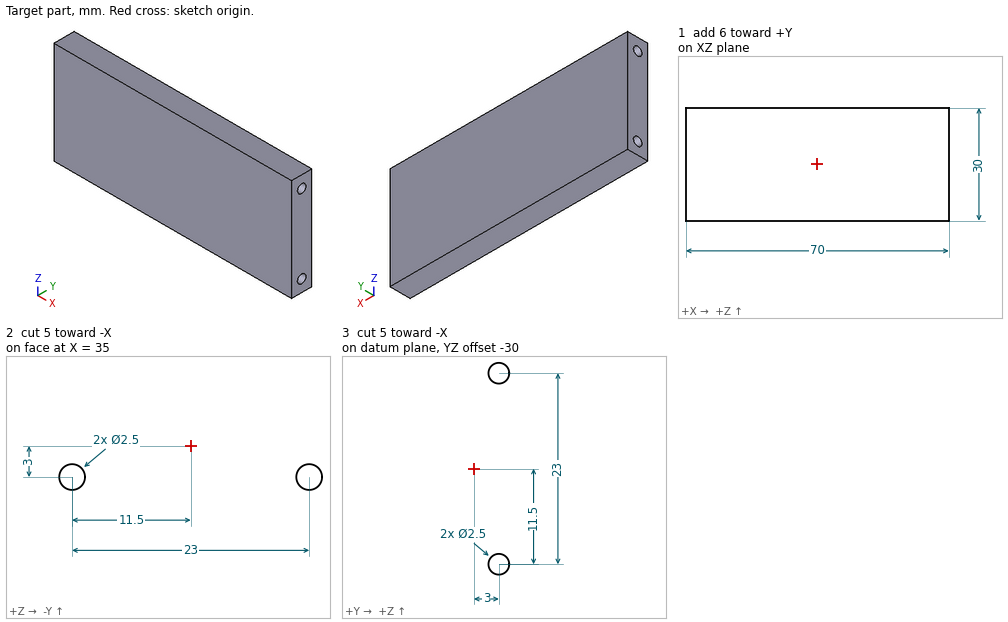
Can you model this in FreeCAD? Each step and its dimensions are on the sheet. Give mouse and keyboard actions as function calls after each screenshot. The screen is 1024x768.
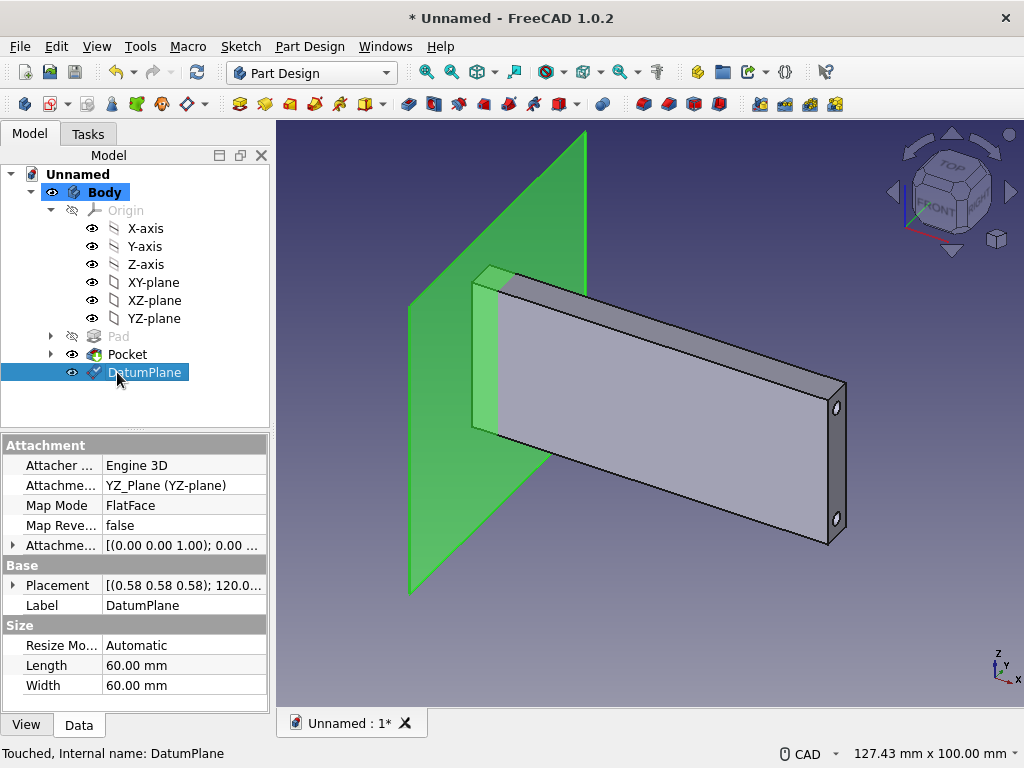
click(50, 104)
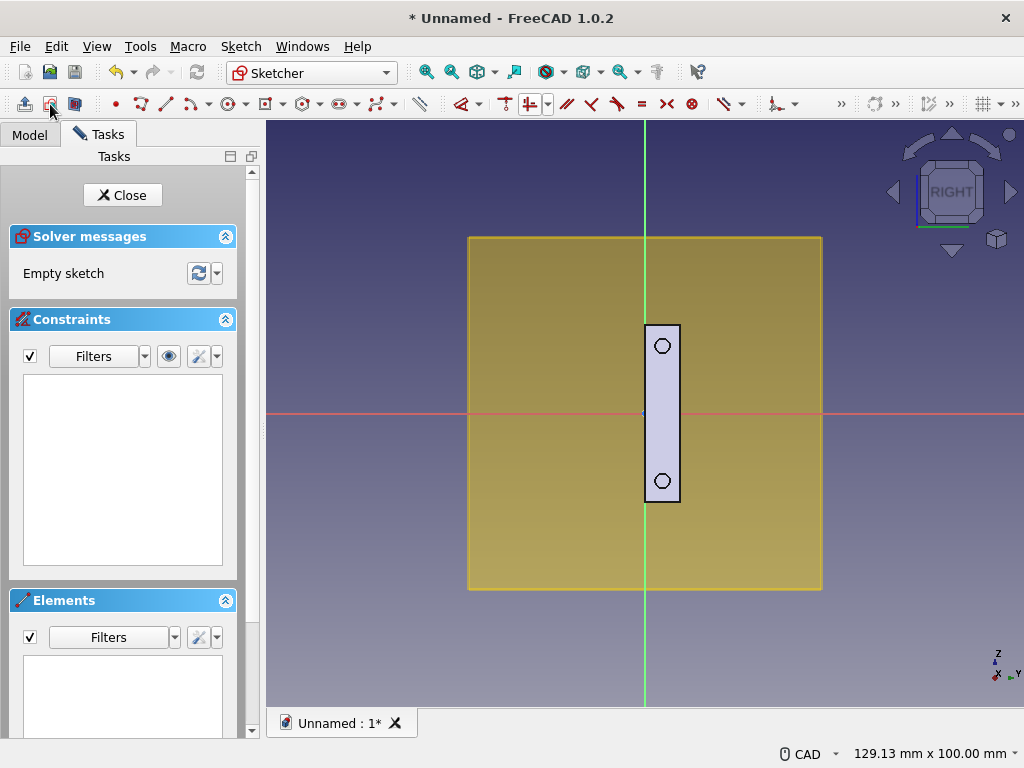
key(q)
key(s)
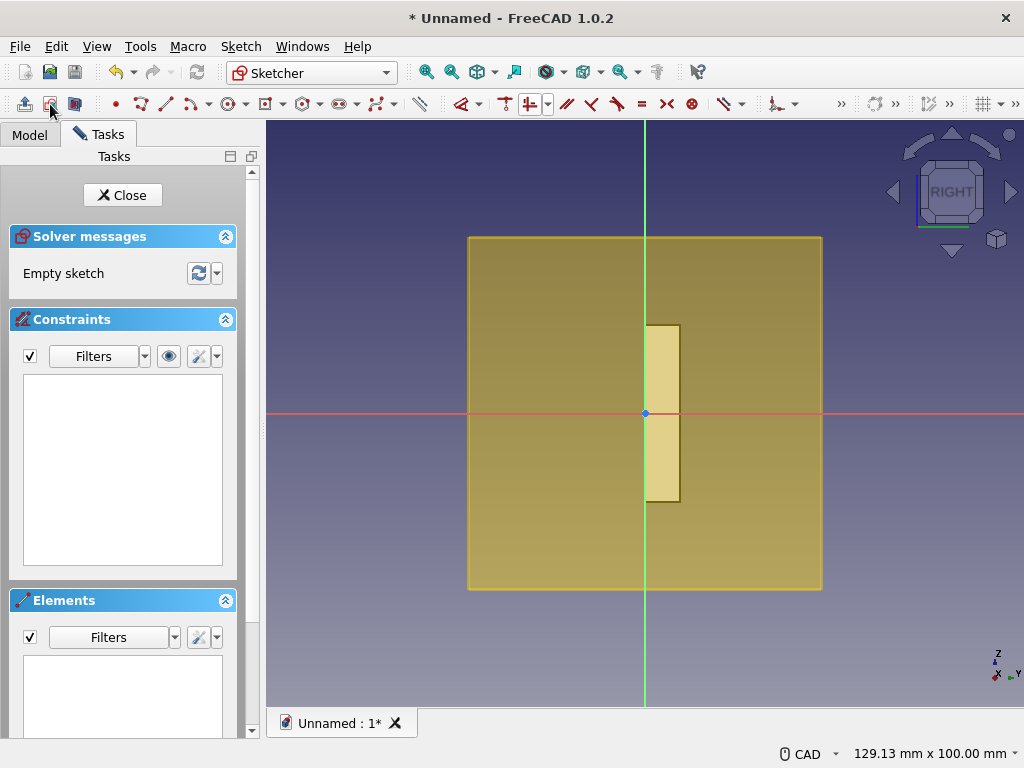
scroll(705, 414, up, 5)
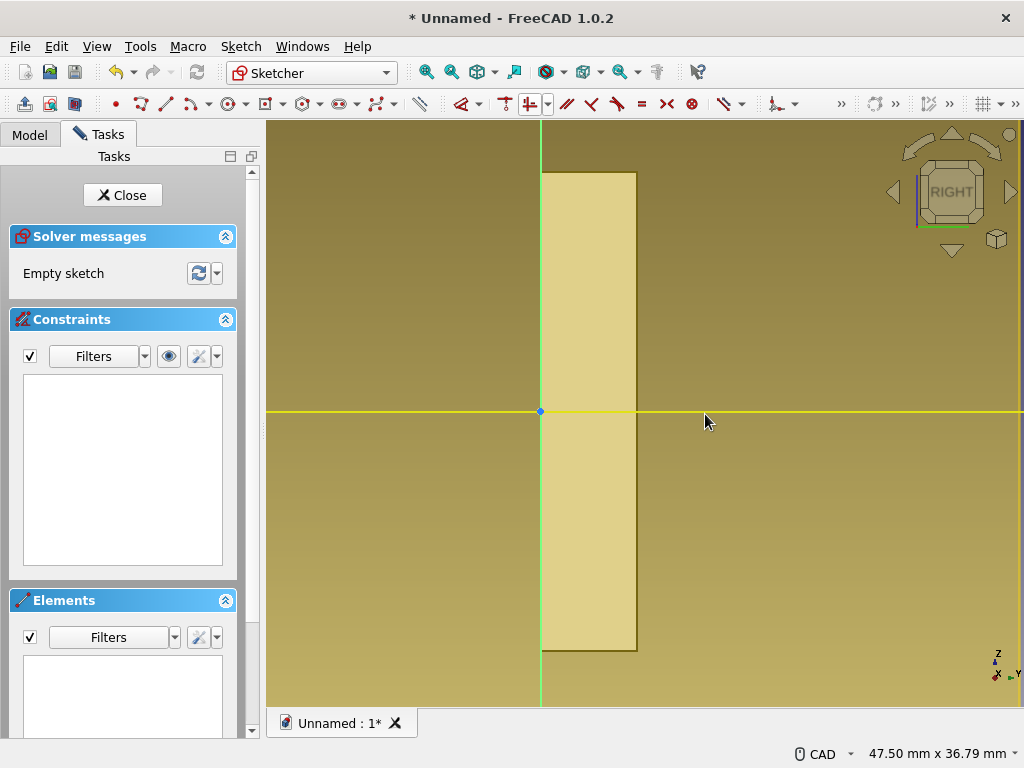
click(228, 104)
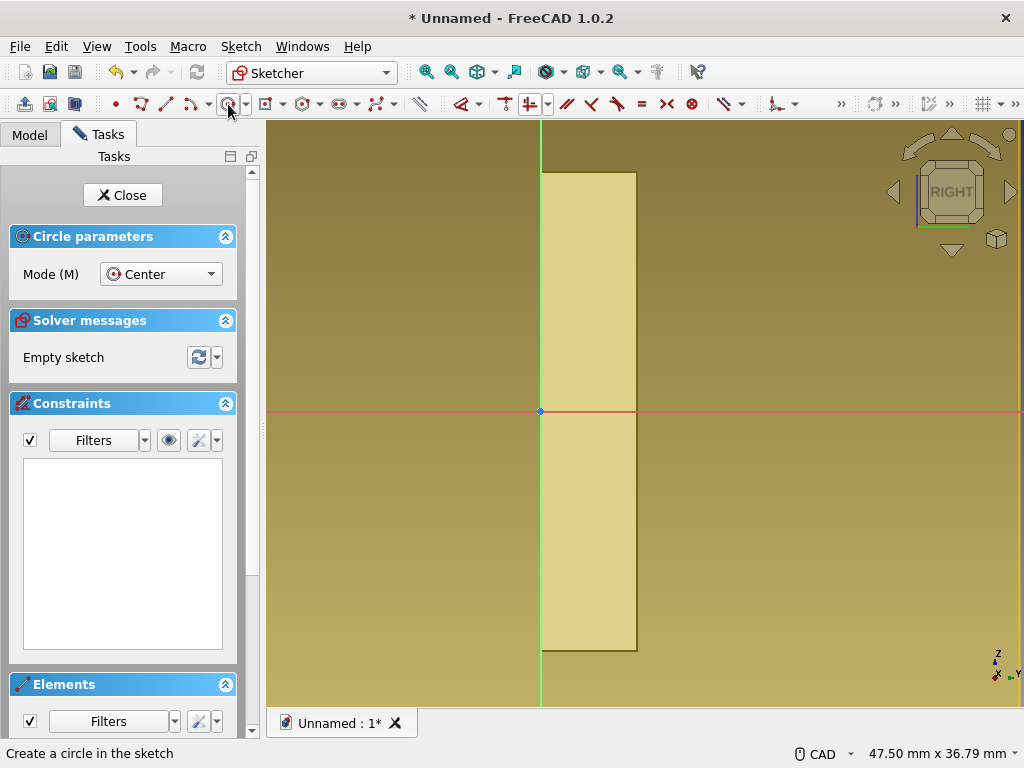
click(589, 595)
click(603, 581)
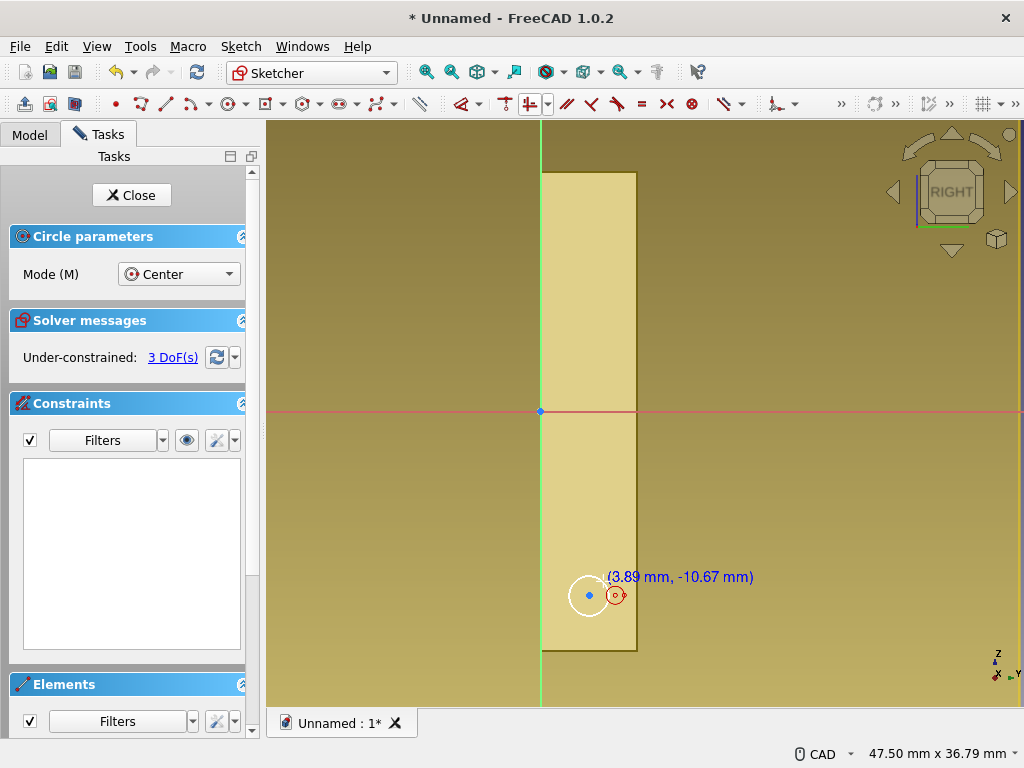
click(589, 228)
click(603, 214)
key(Escape)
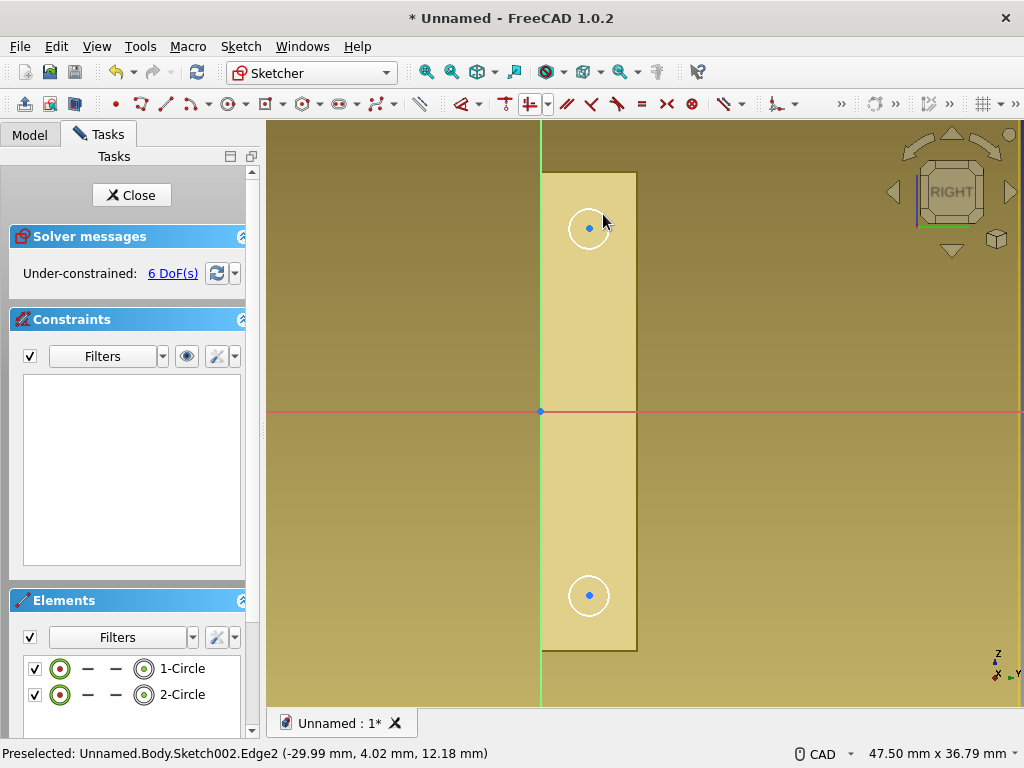
click(603, 582)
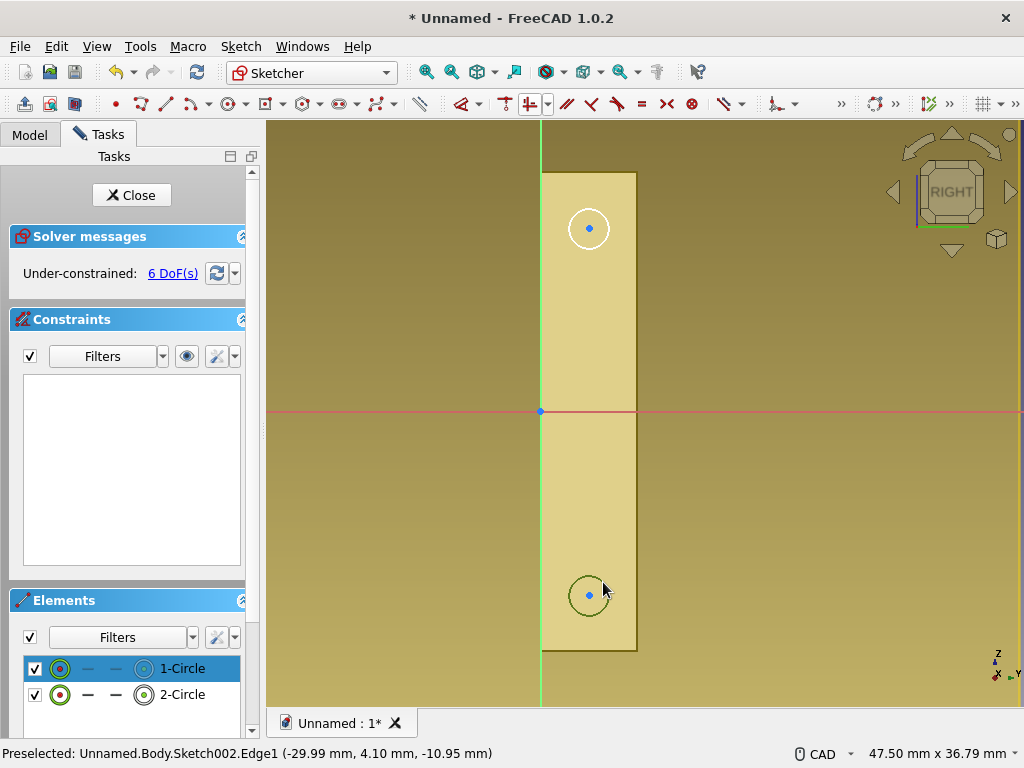
click(603, 215)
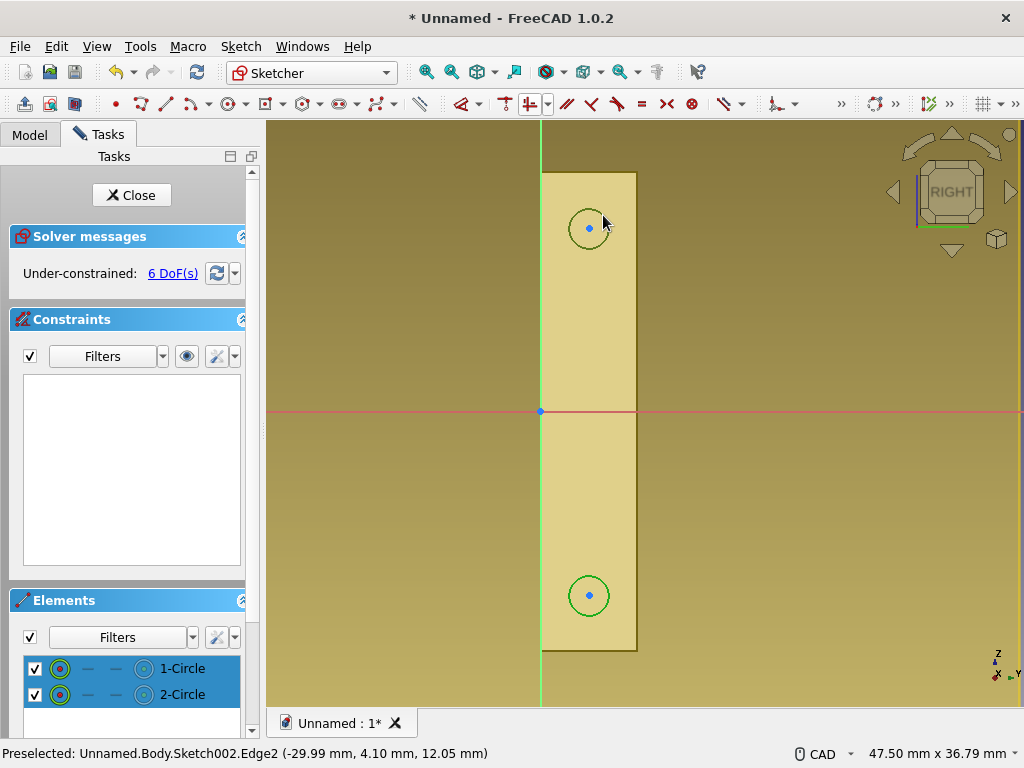
click(642, 104)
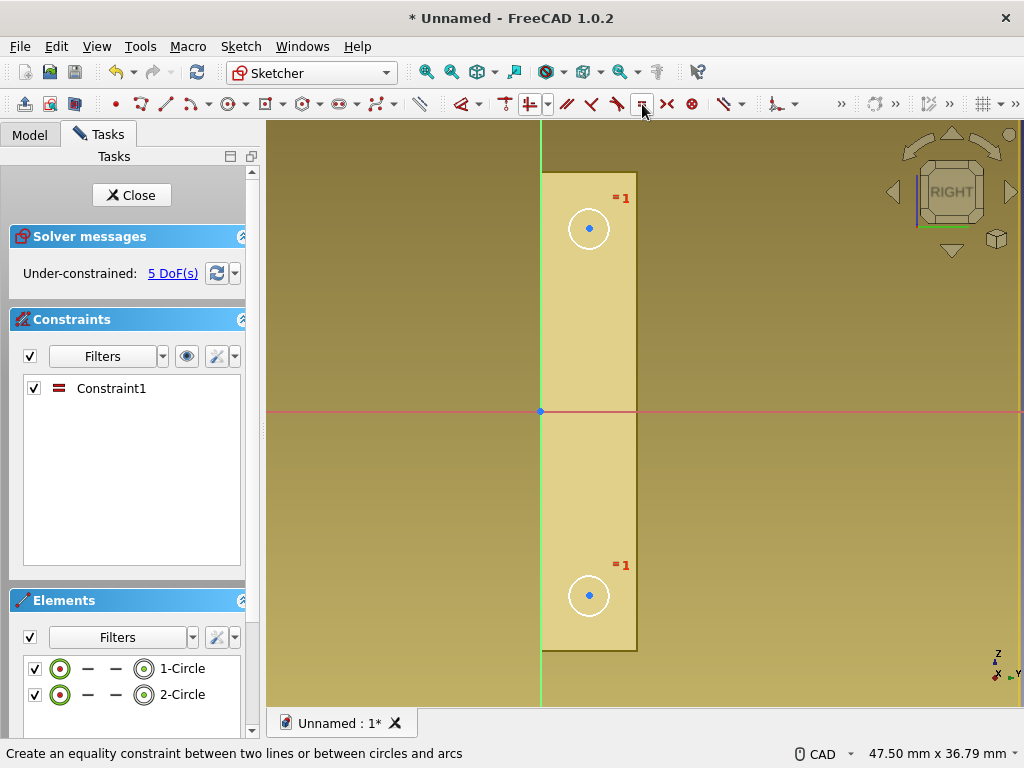
click(589, 596)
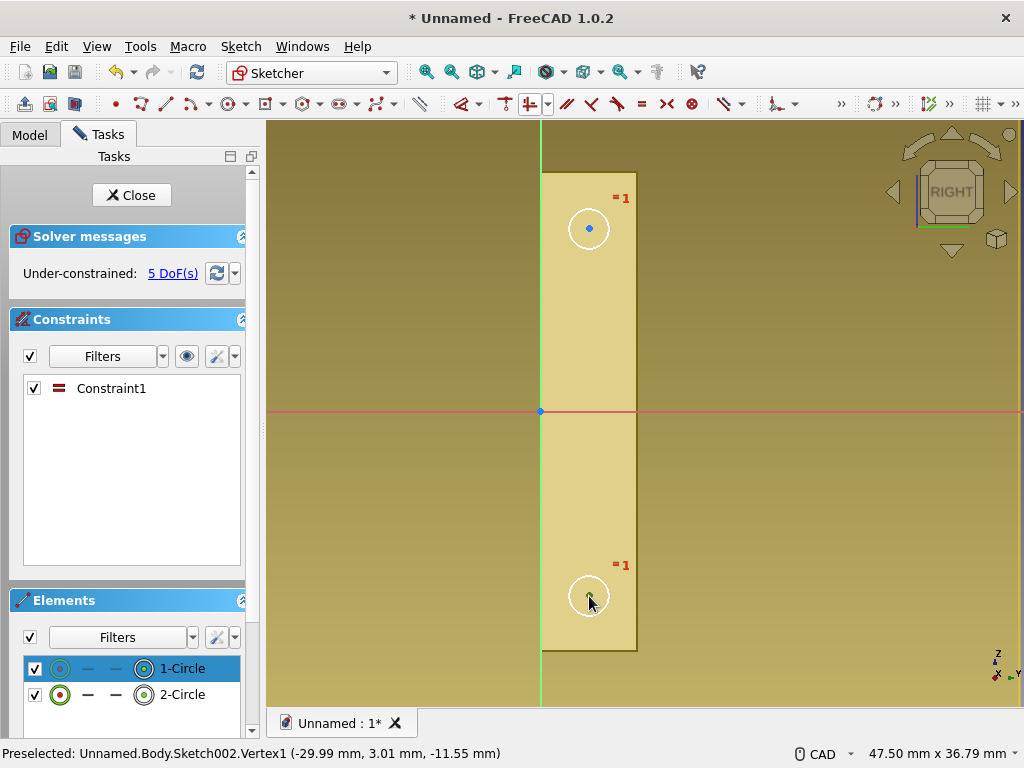
click(589, 229)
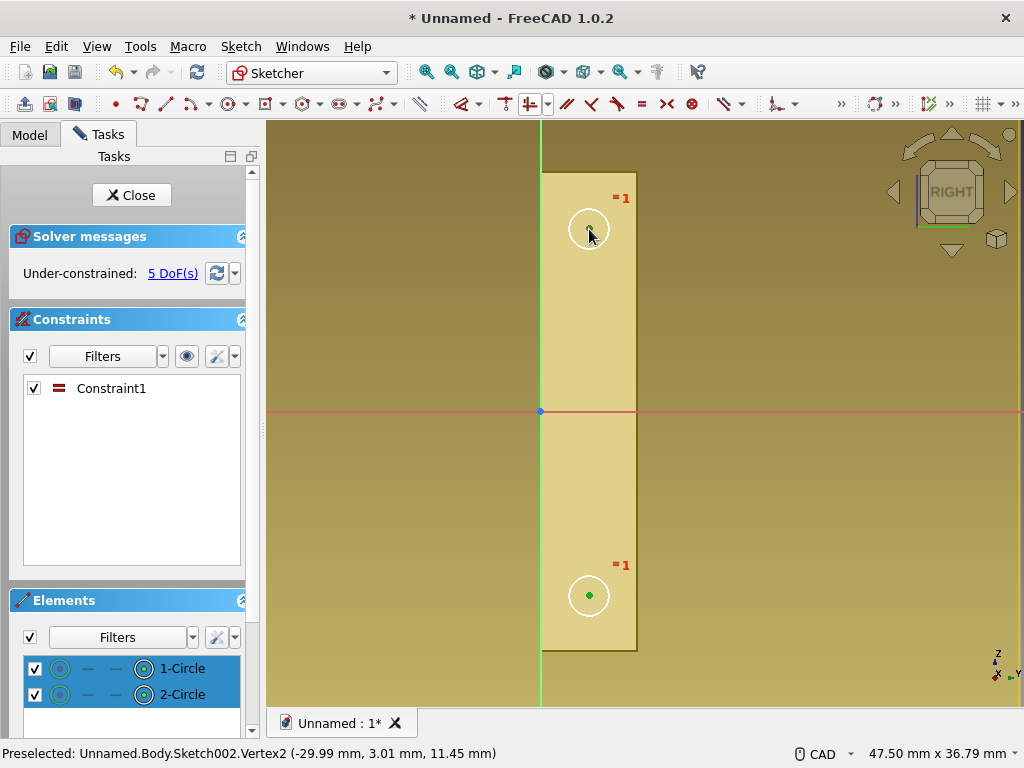
click(548, 104)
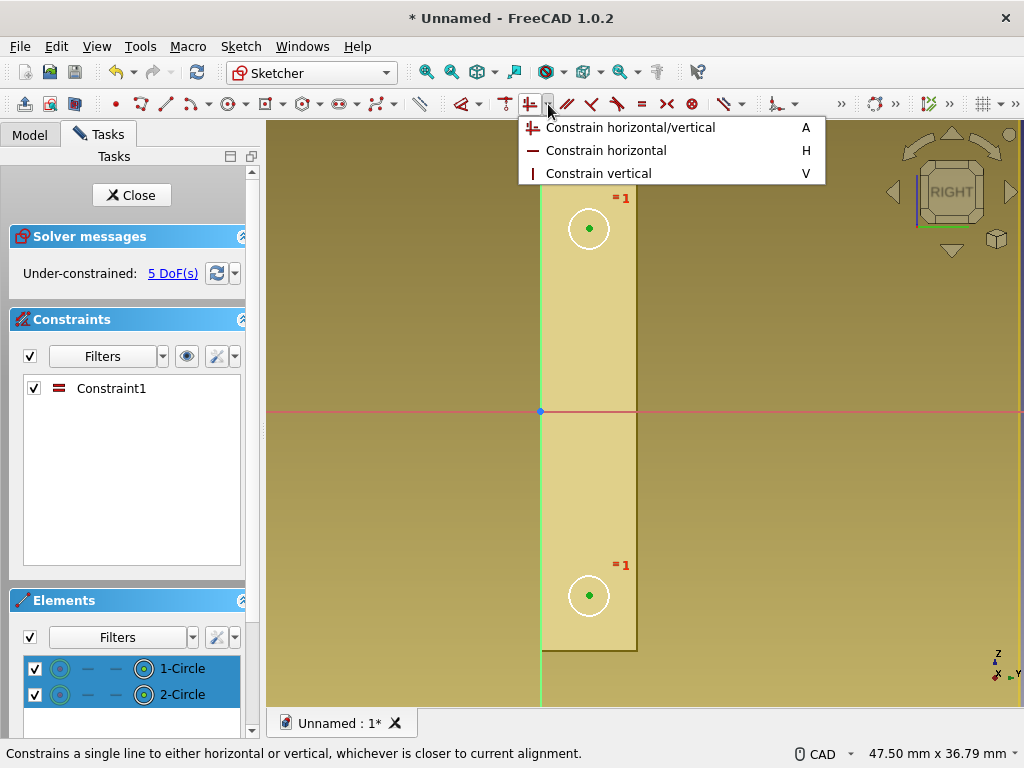
click(672, 174)